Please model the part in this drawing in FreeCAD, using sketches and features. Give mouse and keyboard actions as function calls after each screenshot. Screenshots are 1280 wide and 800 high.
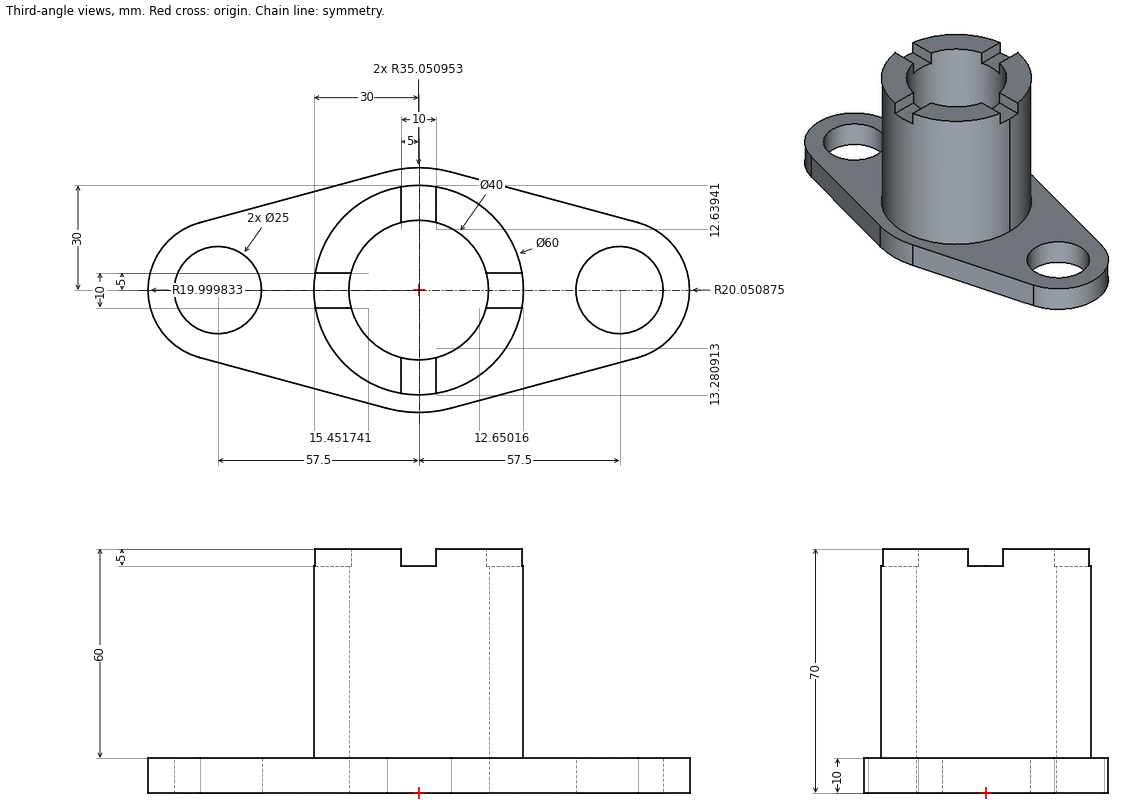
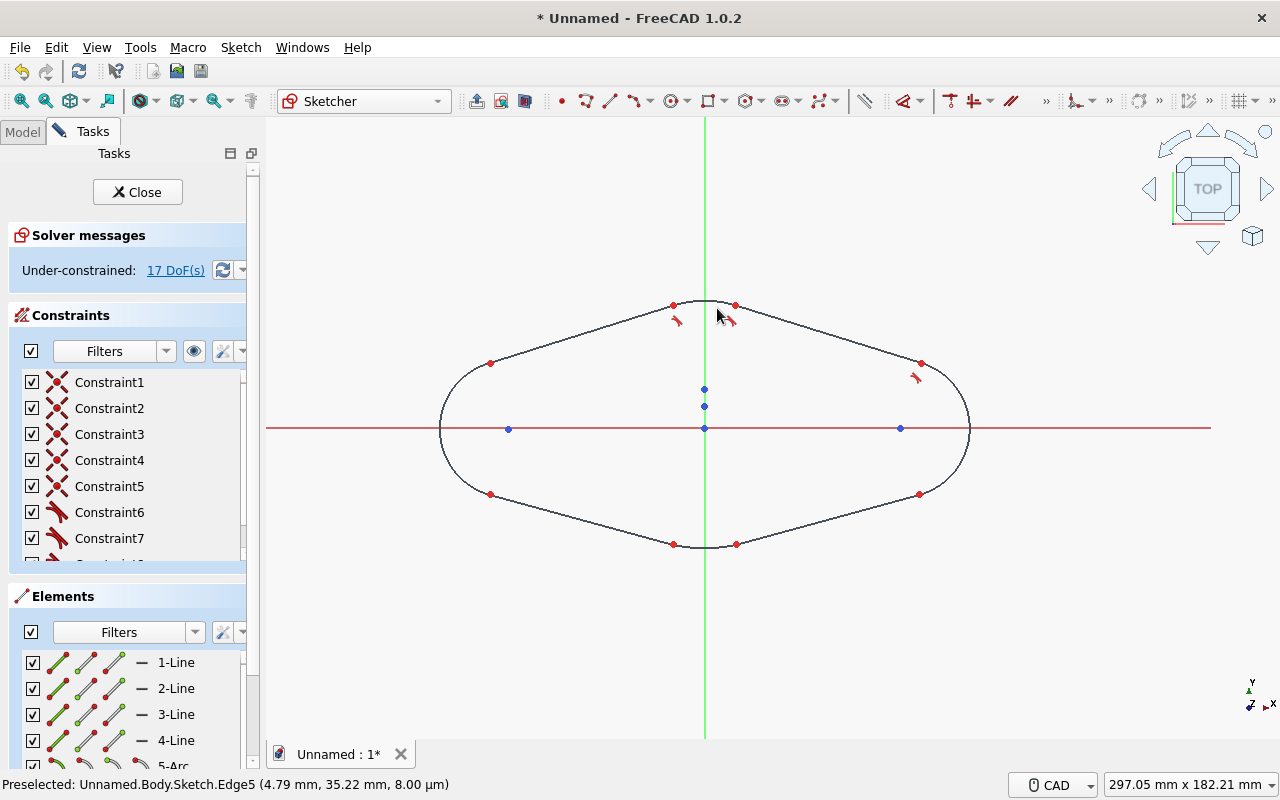
click(618, 323)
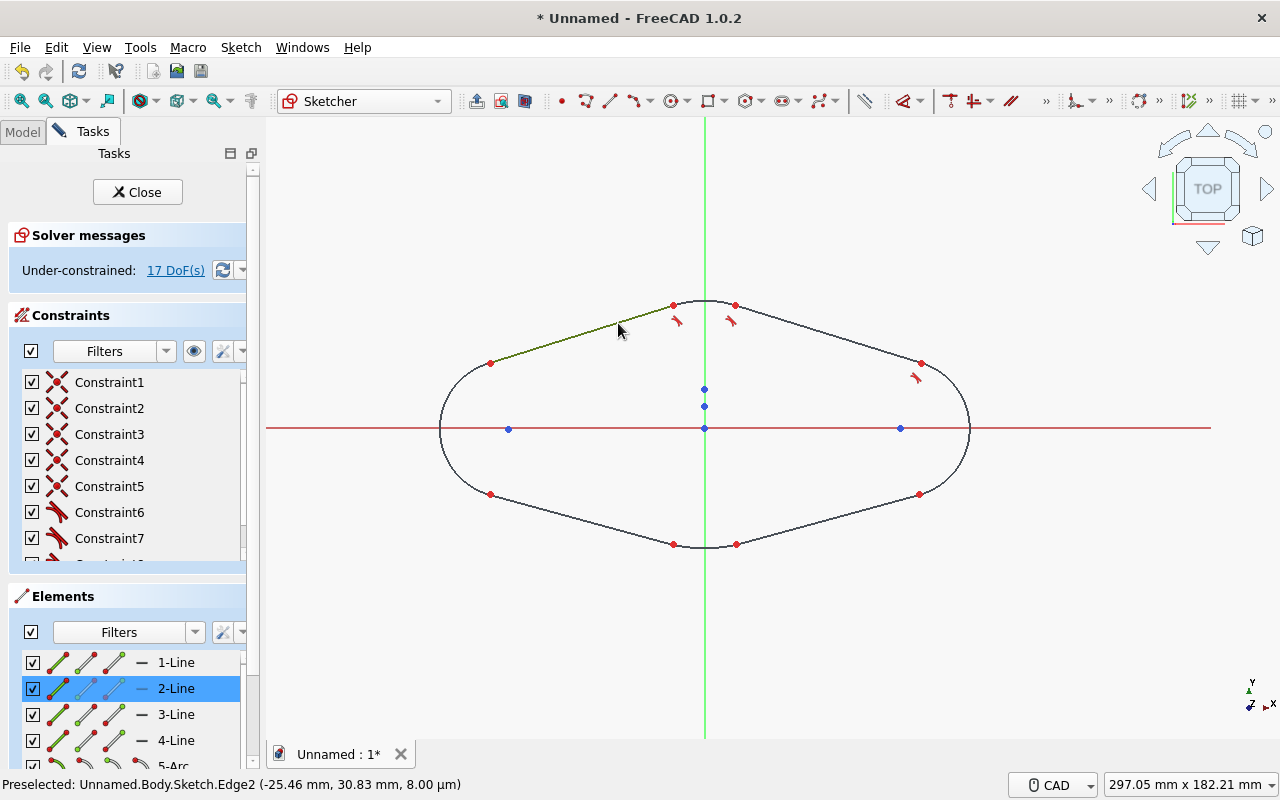
click(449, 395)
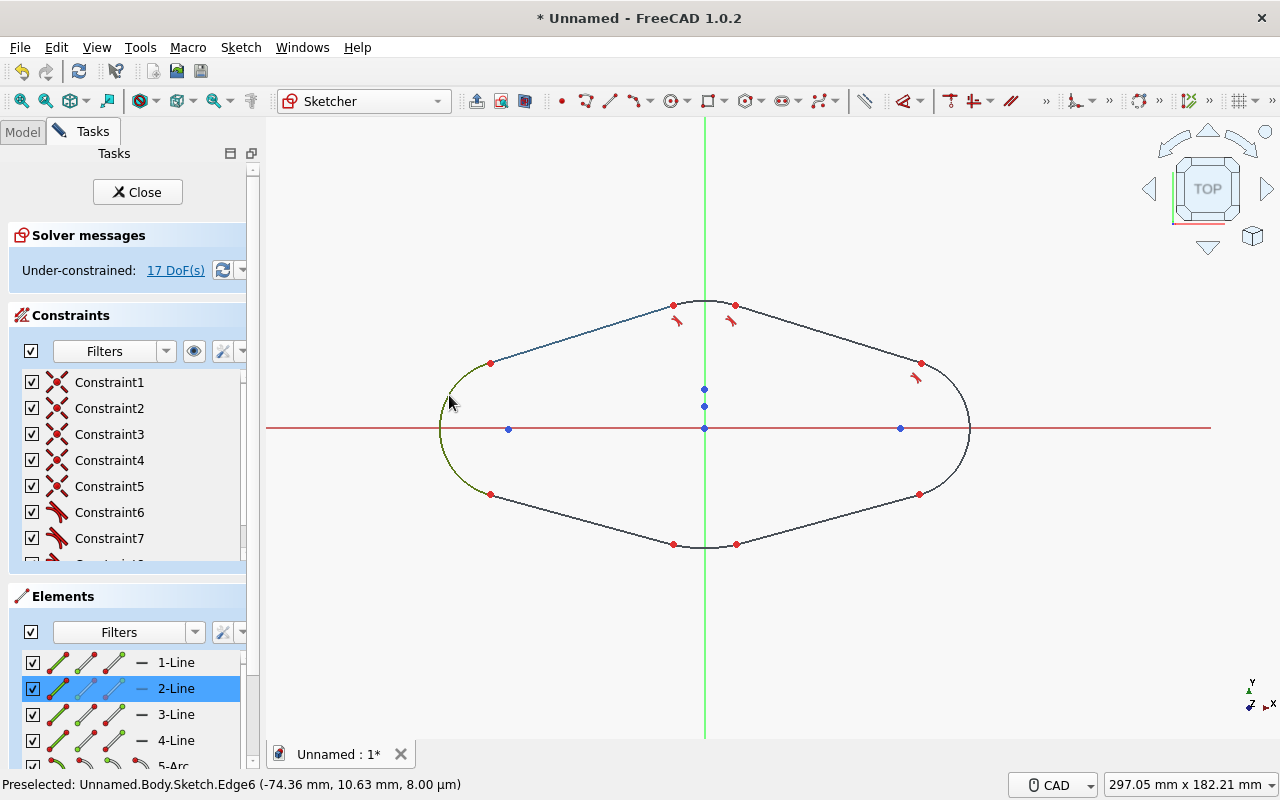
key(t)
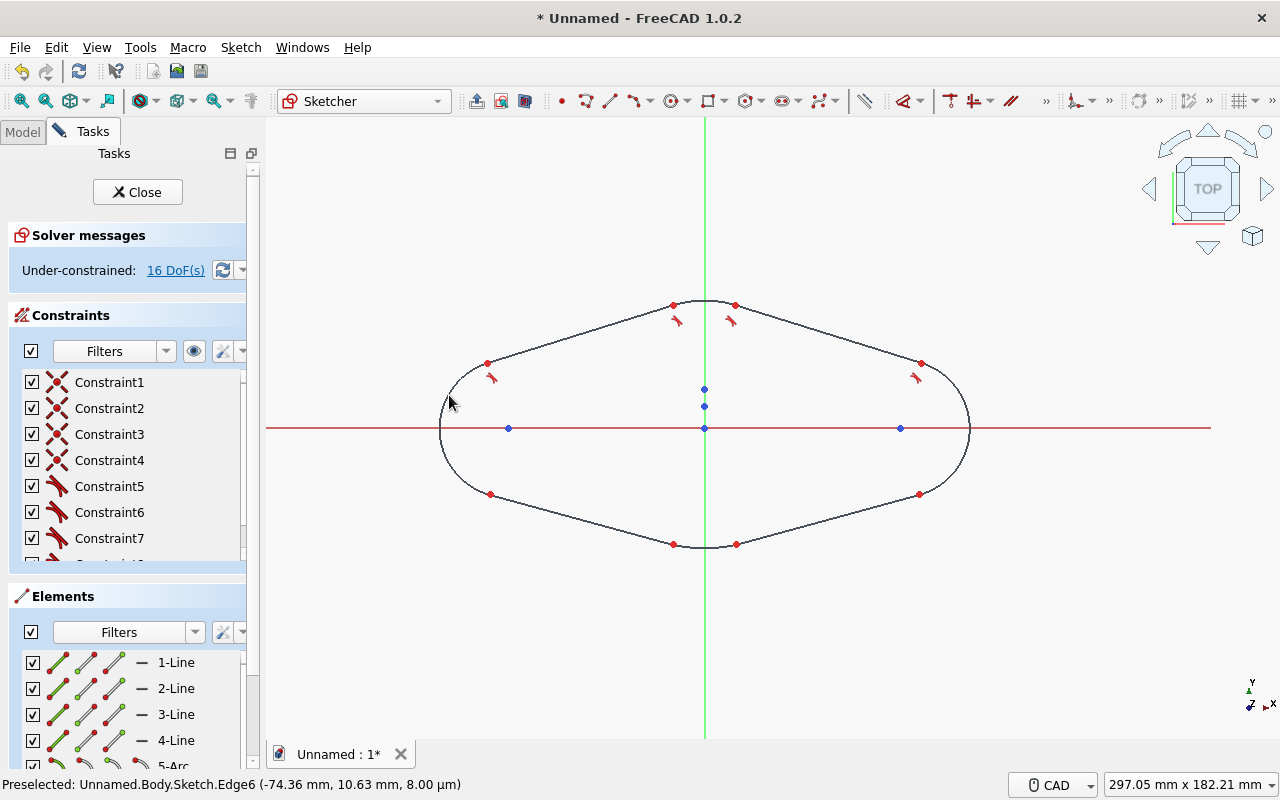
click(545, 510)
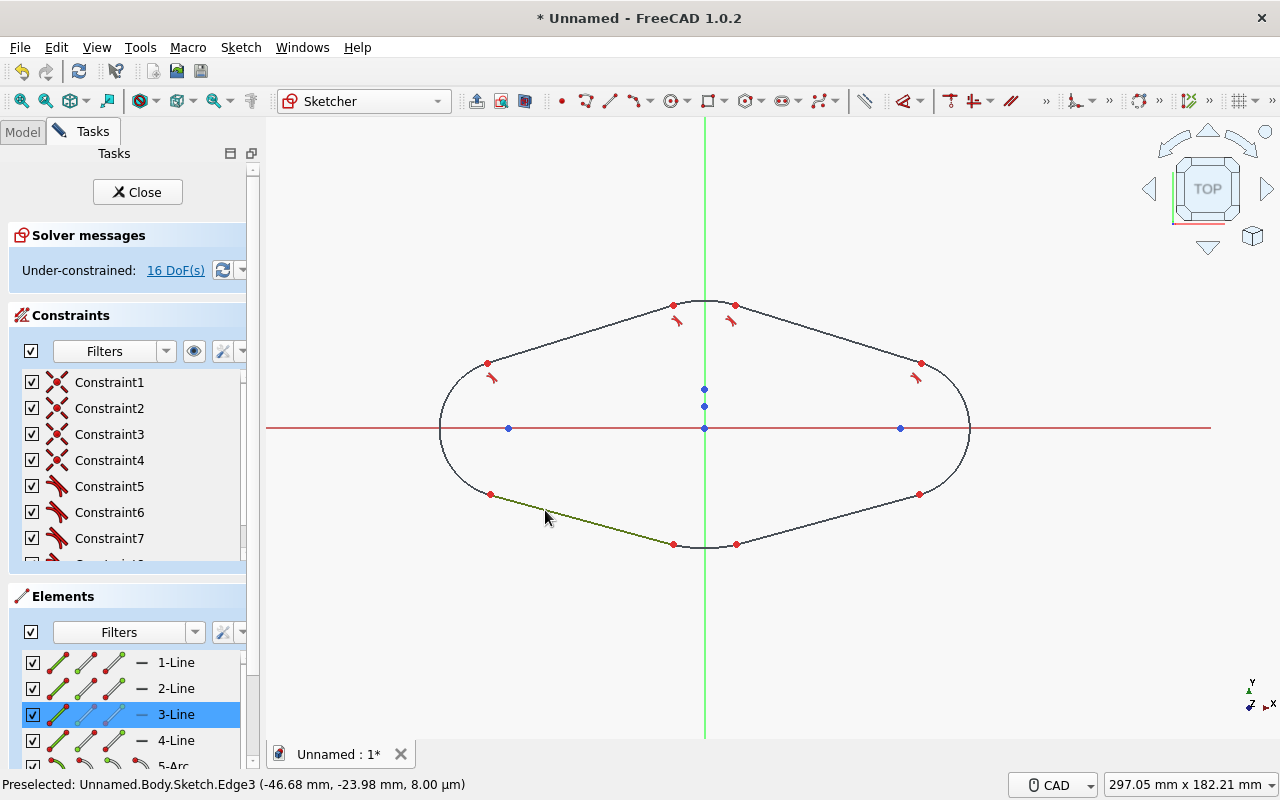
click(448, 396)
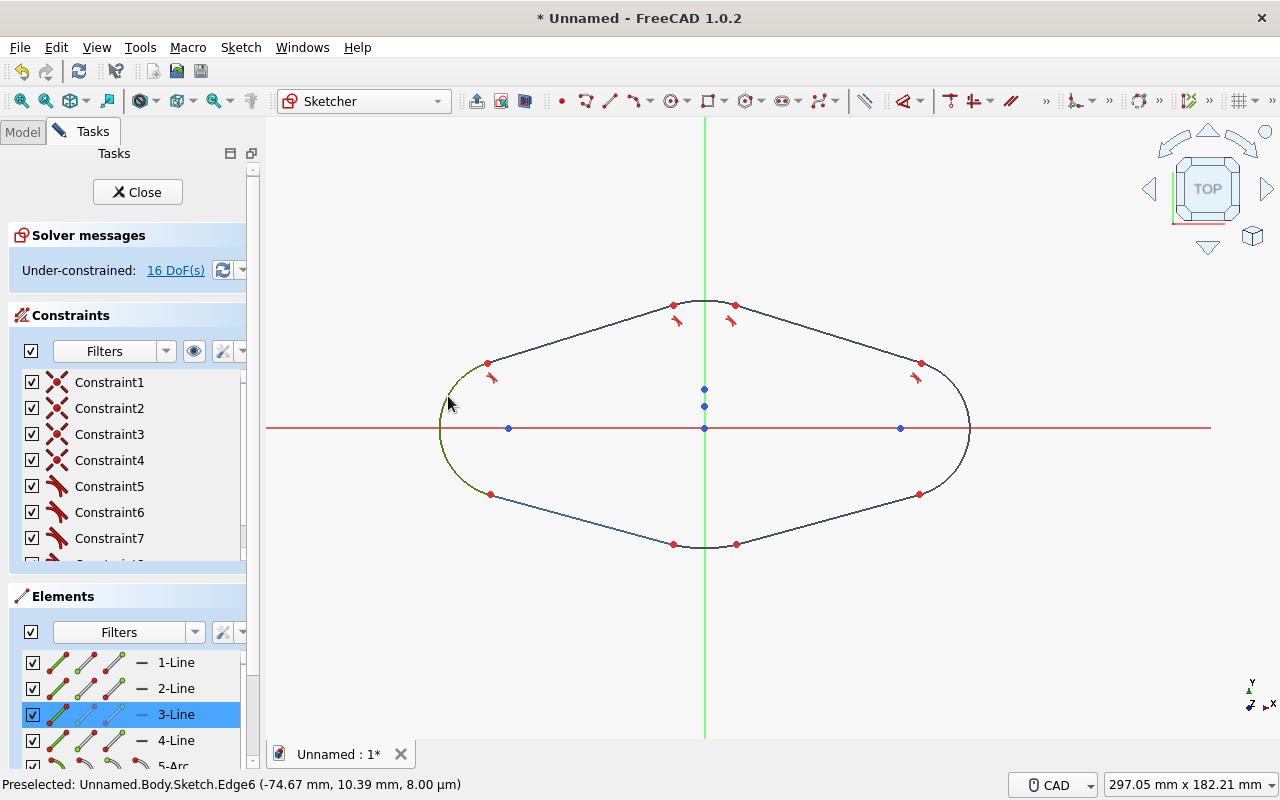
key(t)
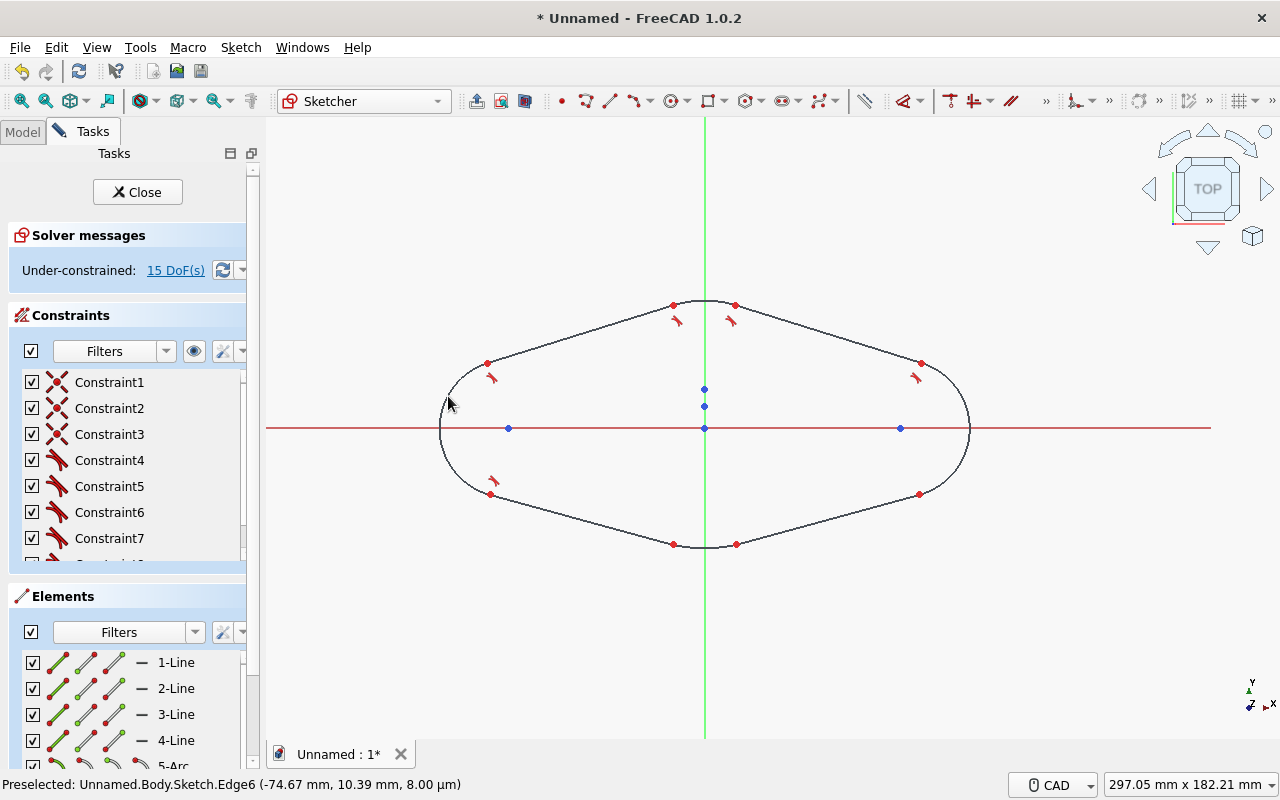
click(545, 510)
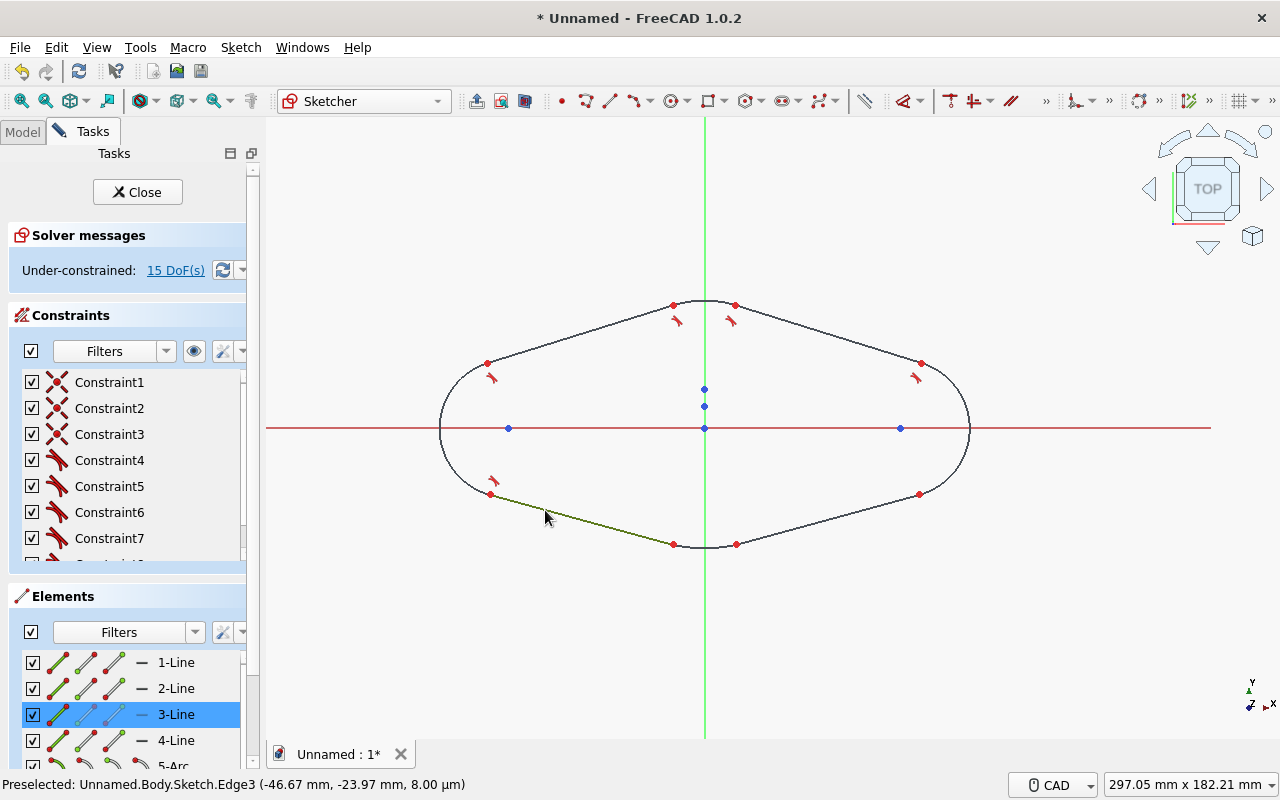
click(692, 548)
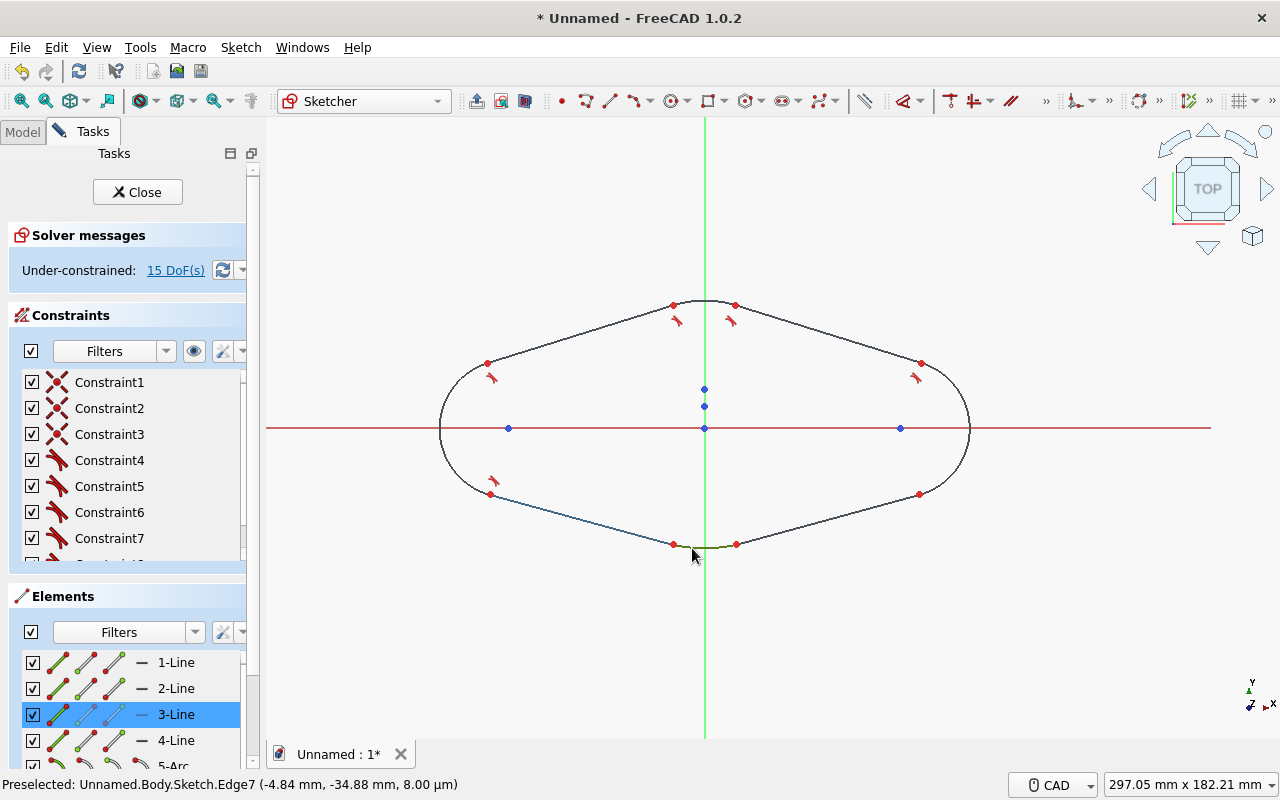
key(t)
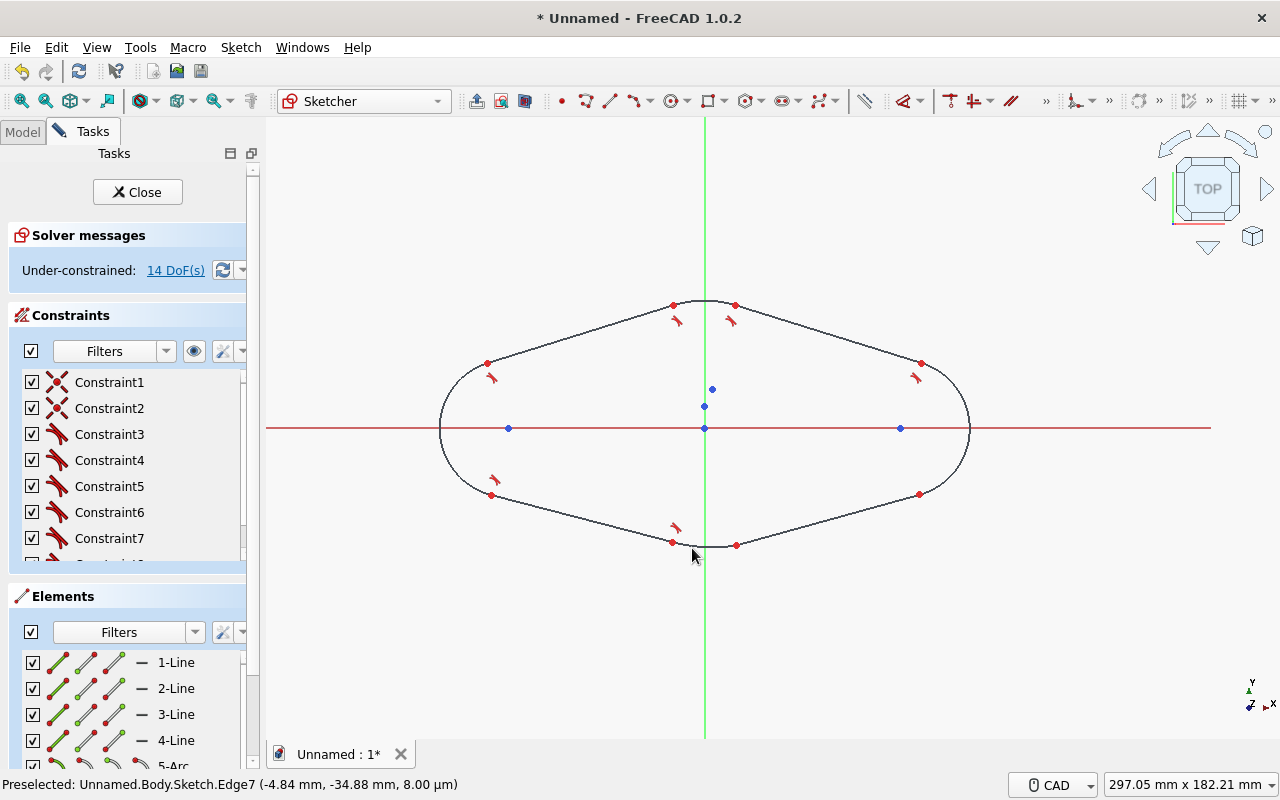
click(791, 530)